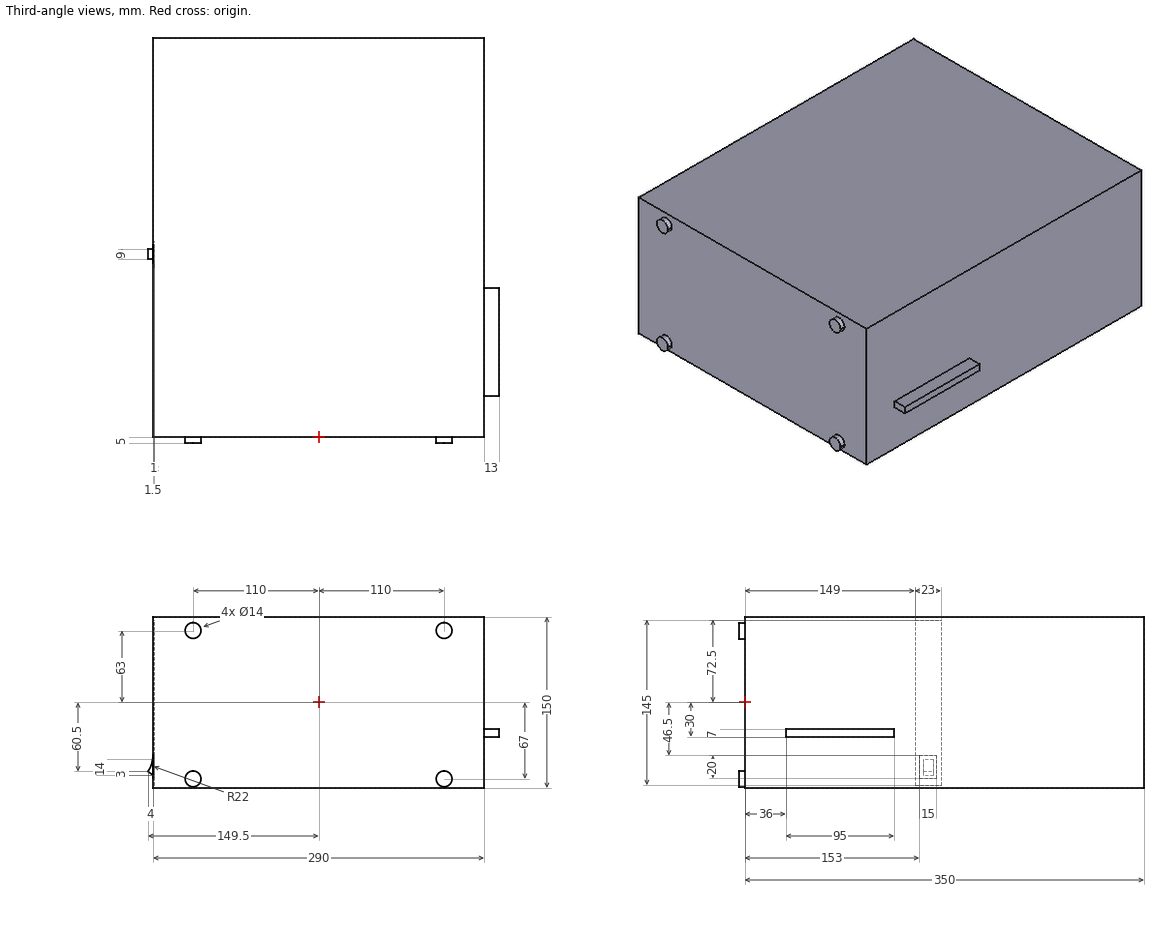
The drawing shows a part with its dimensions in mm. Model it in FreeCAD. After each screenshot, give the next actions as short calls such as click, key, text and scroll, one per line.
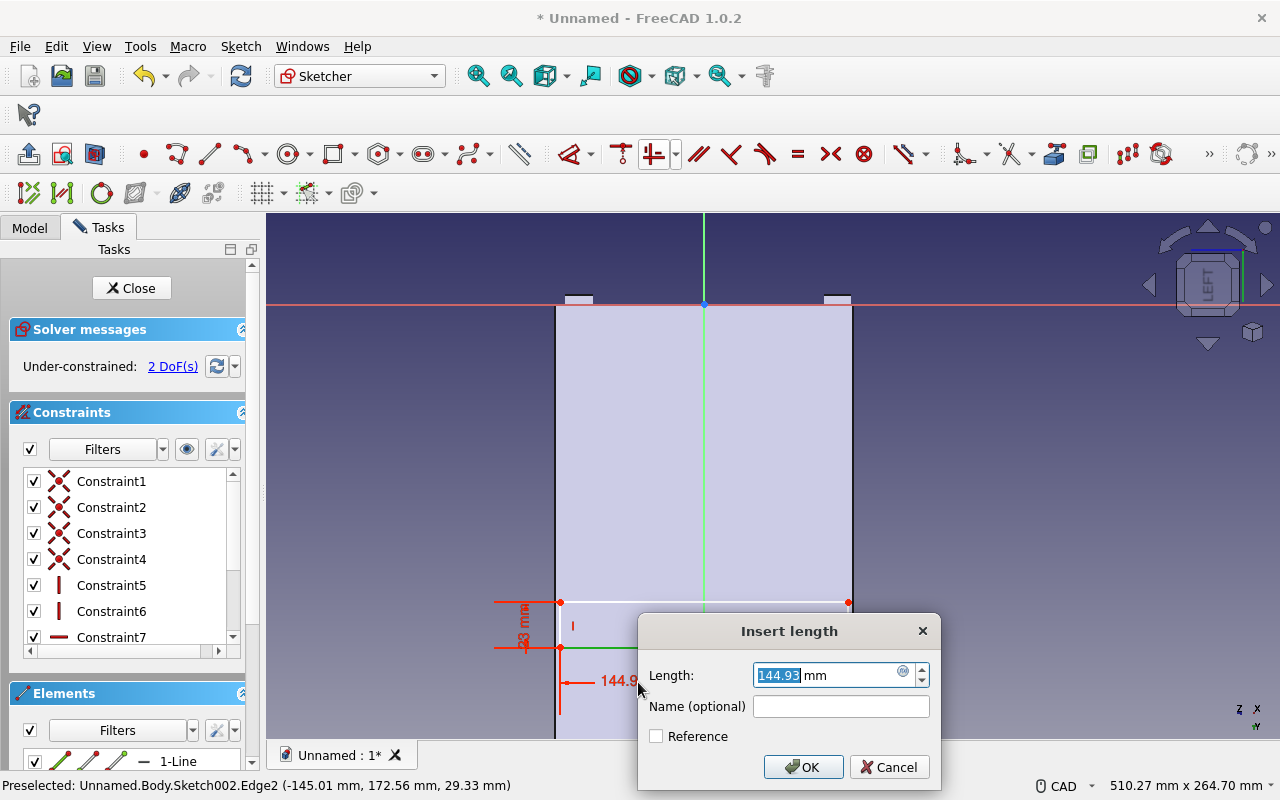
text(145)
key(Return)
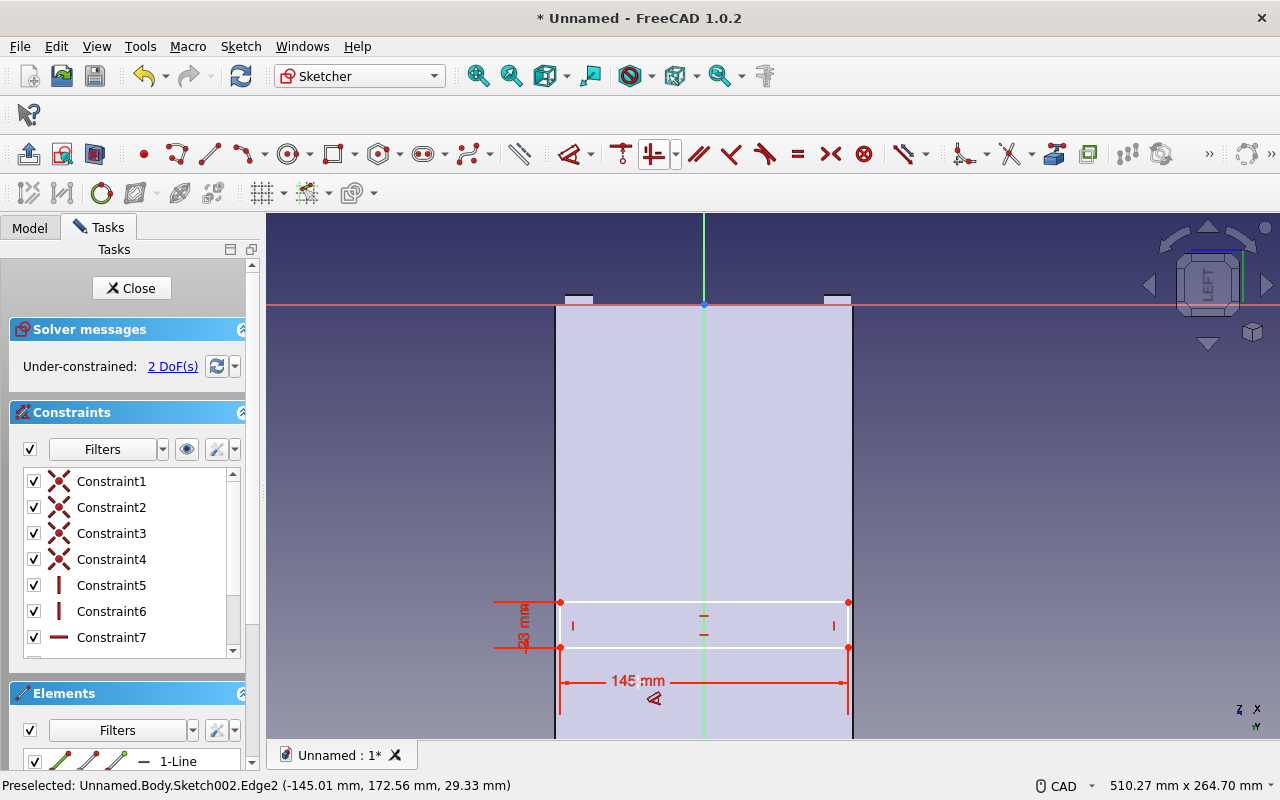
click(560, 602)
click(526, 454)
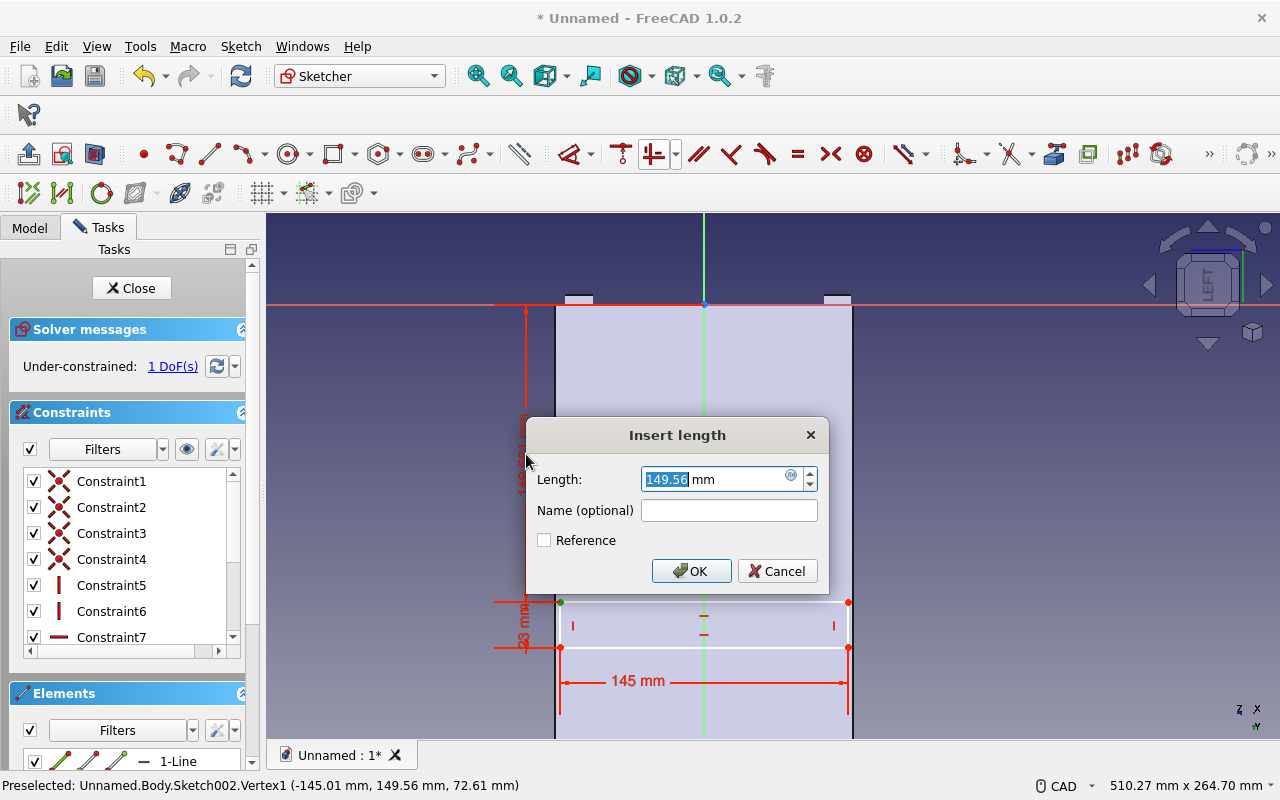
text(149)
key(Return)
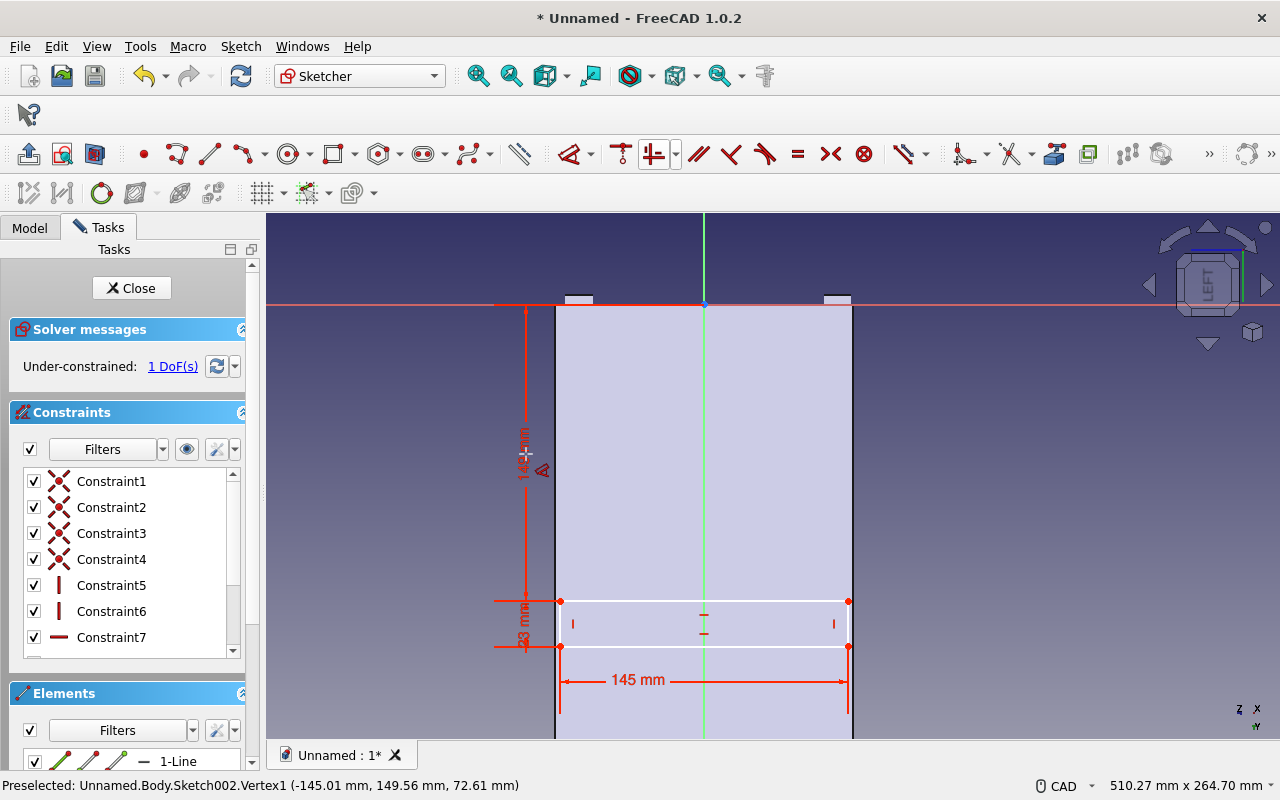
click(560, 601)
click(632, 271)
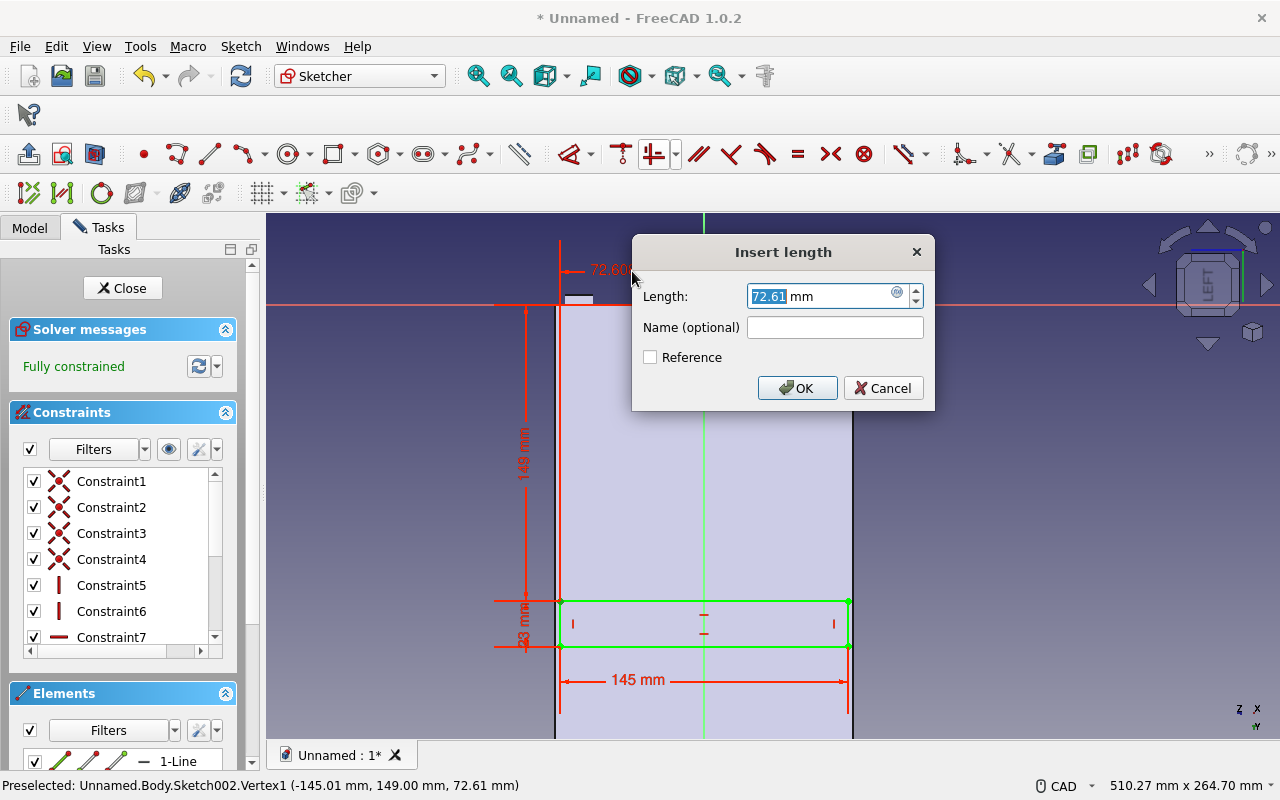
text(72.5)
key(Return)
key(Escape)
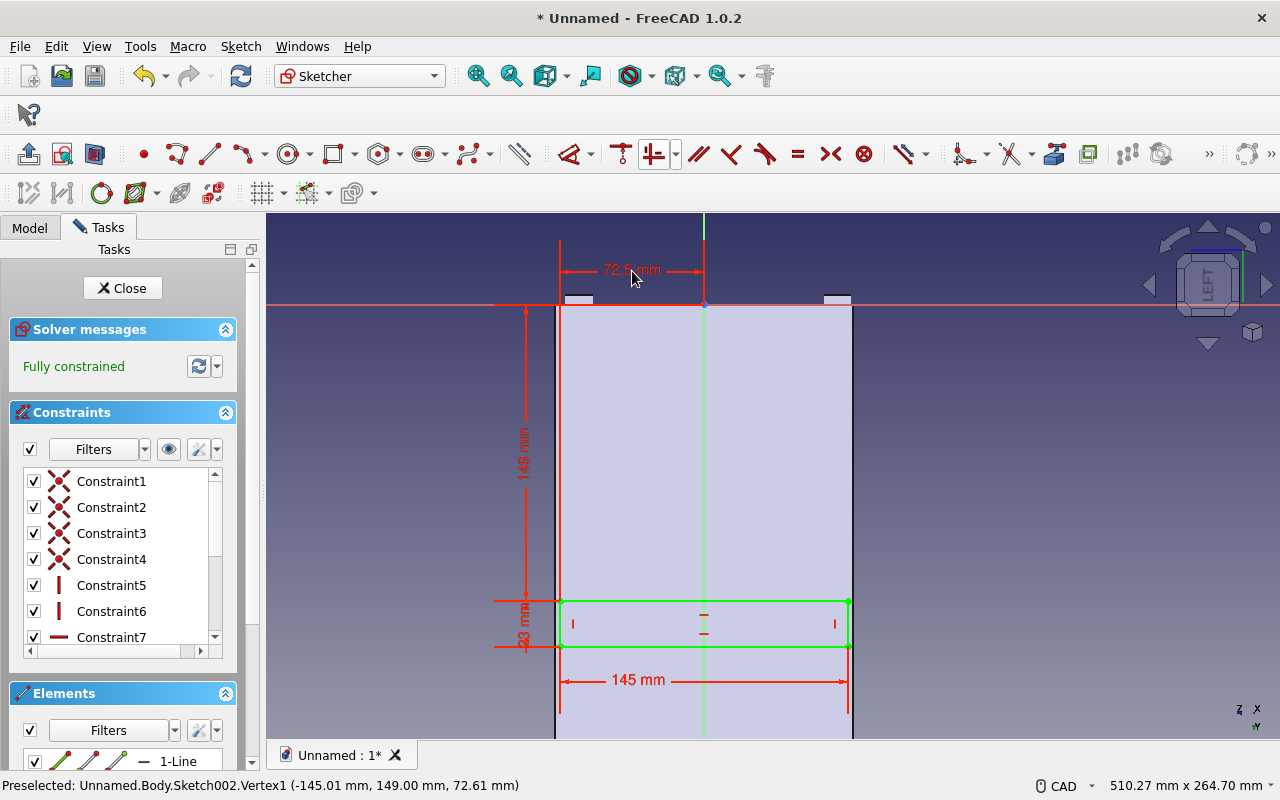
click(123, 288)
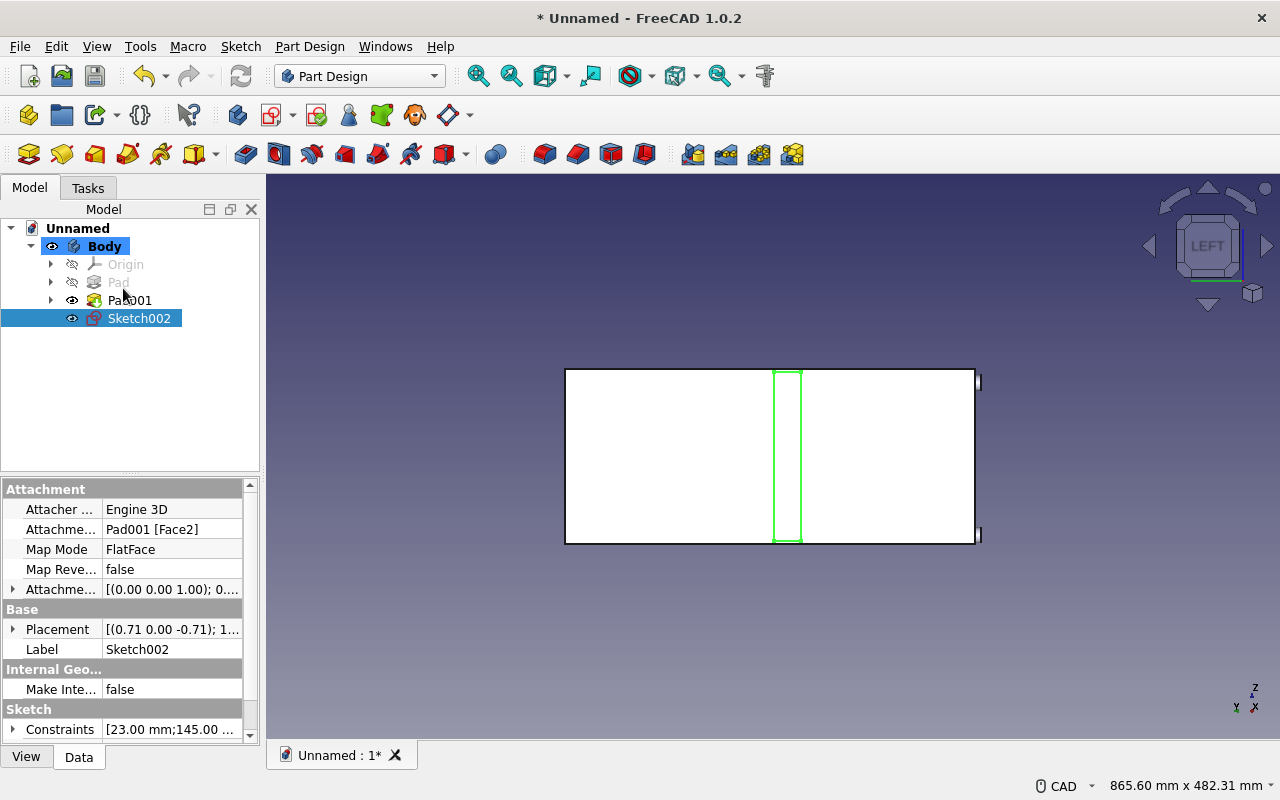
click(246, 154)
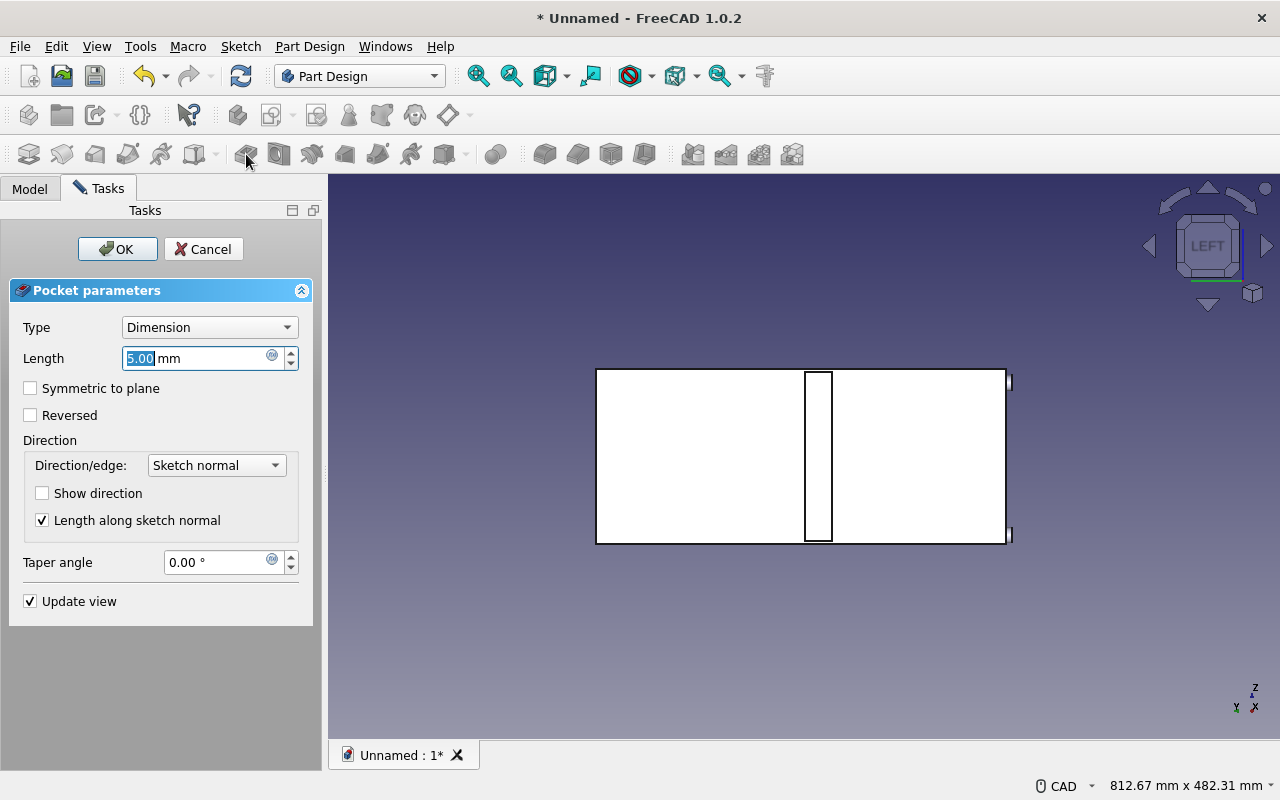
text(1)
key(Tab)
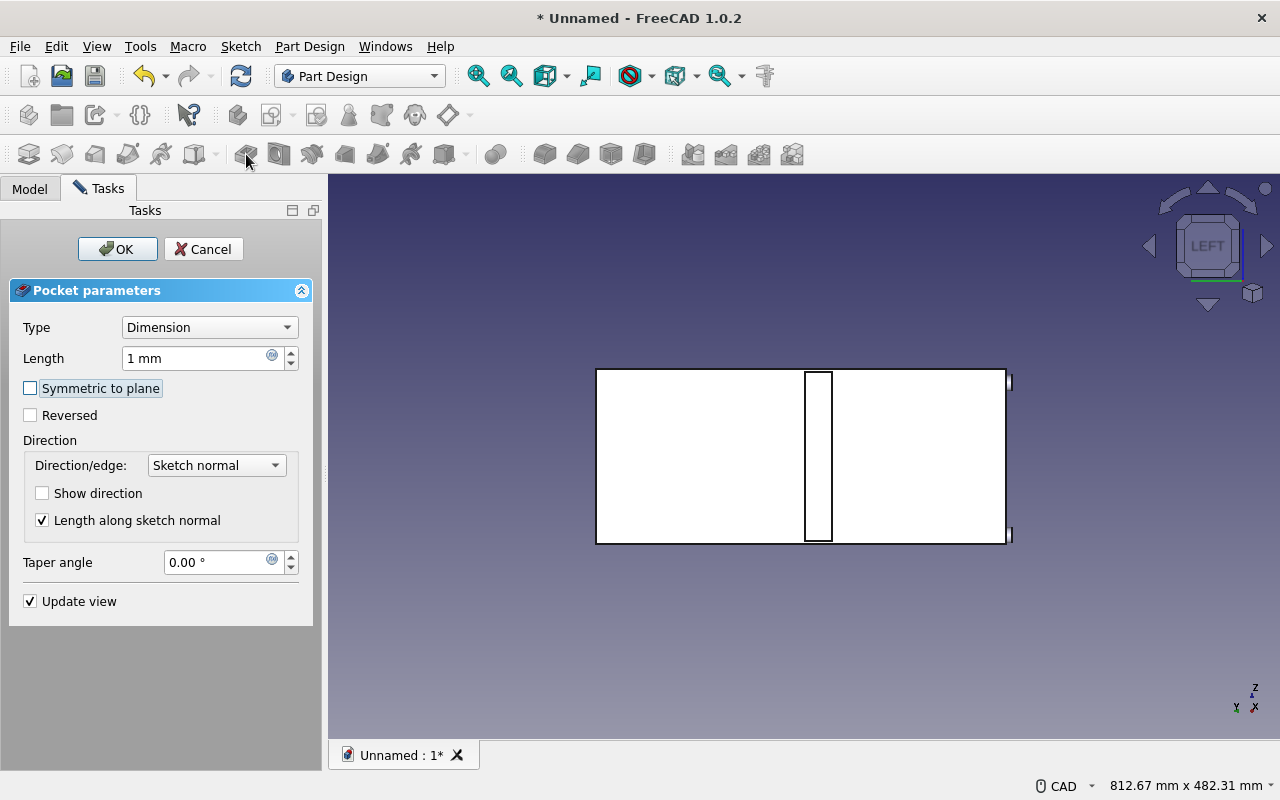
click(118, 249)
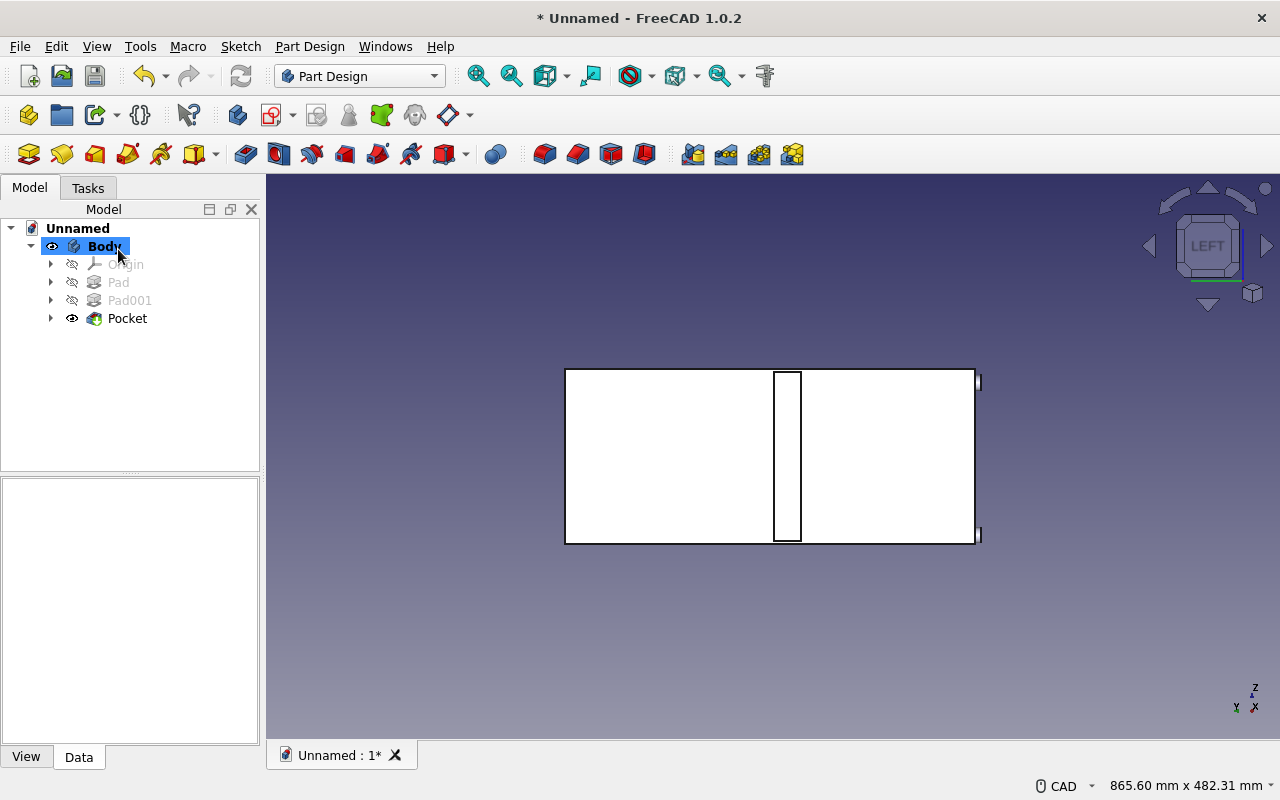
click(479, 76)